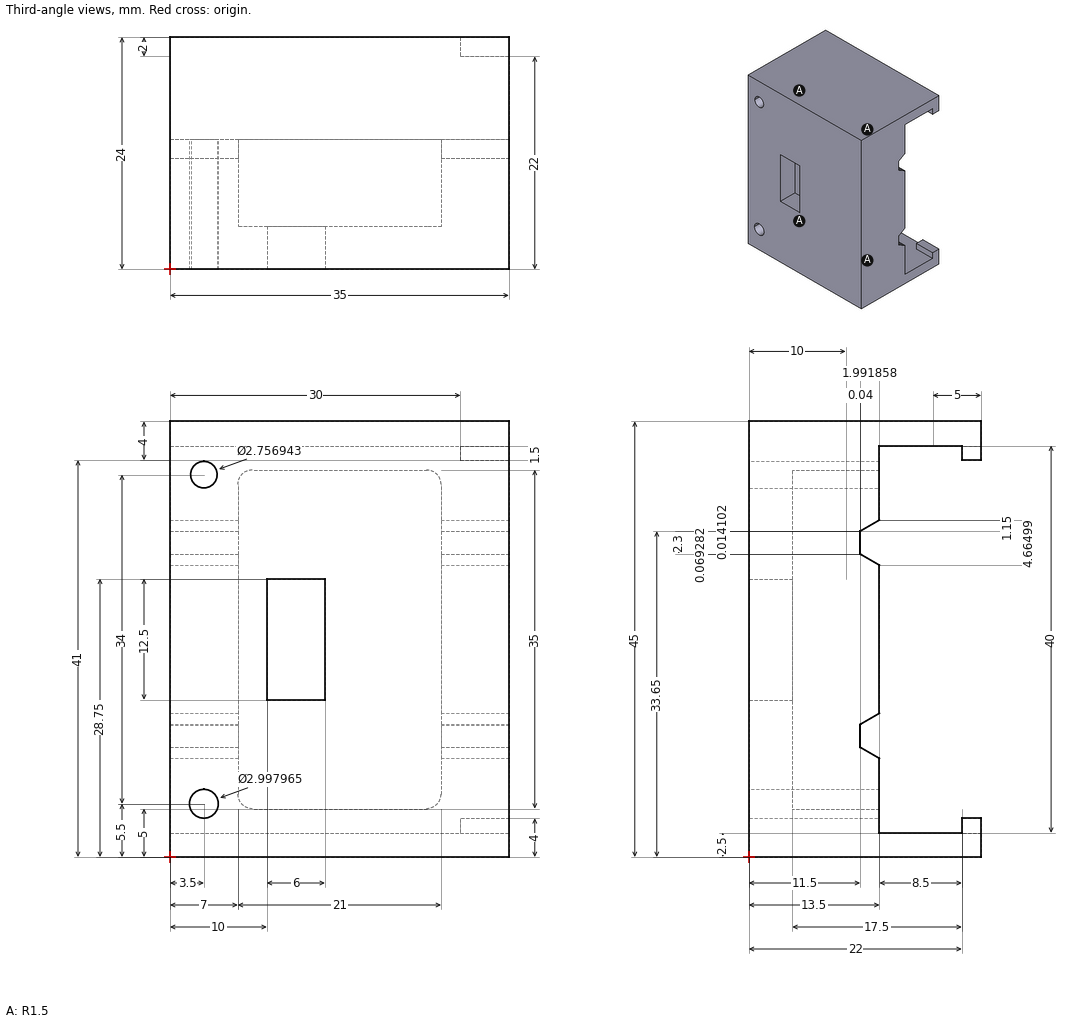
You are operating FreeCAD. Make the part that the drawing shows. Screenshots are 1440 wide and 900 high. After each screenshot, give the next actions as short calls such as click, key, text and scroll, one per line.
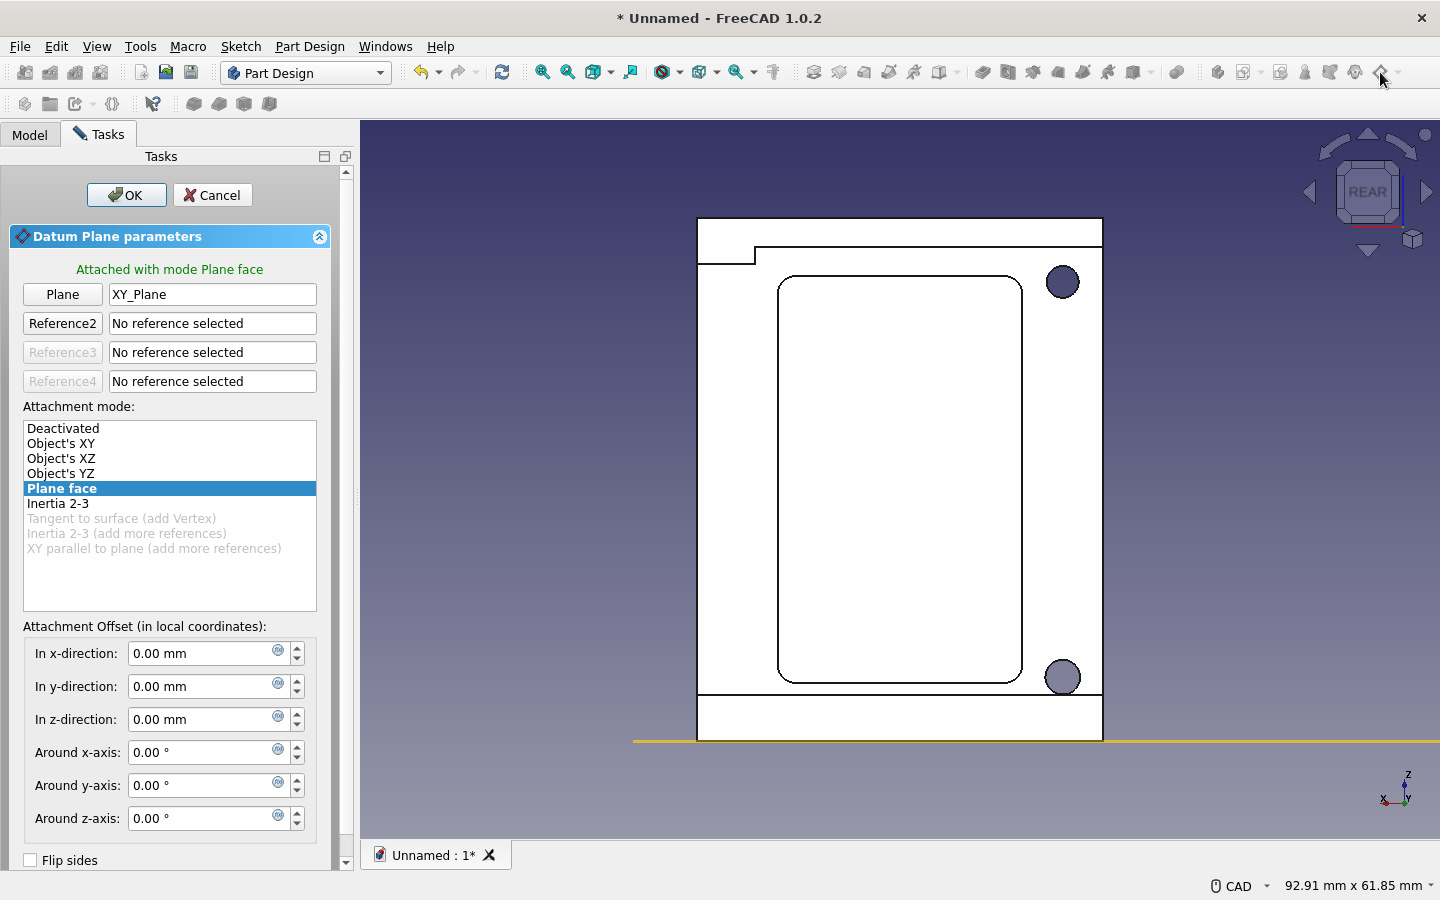
triple_click(210, 720)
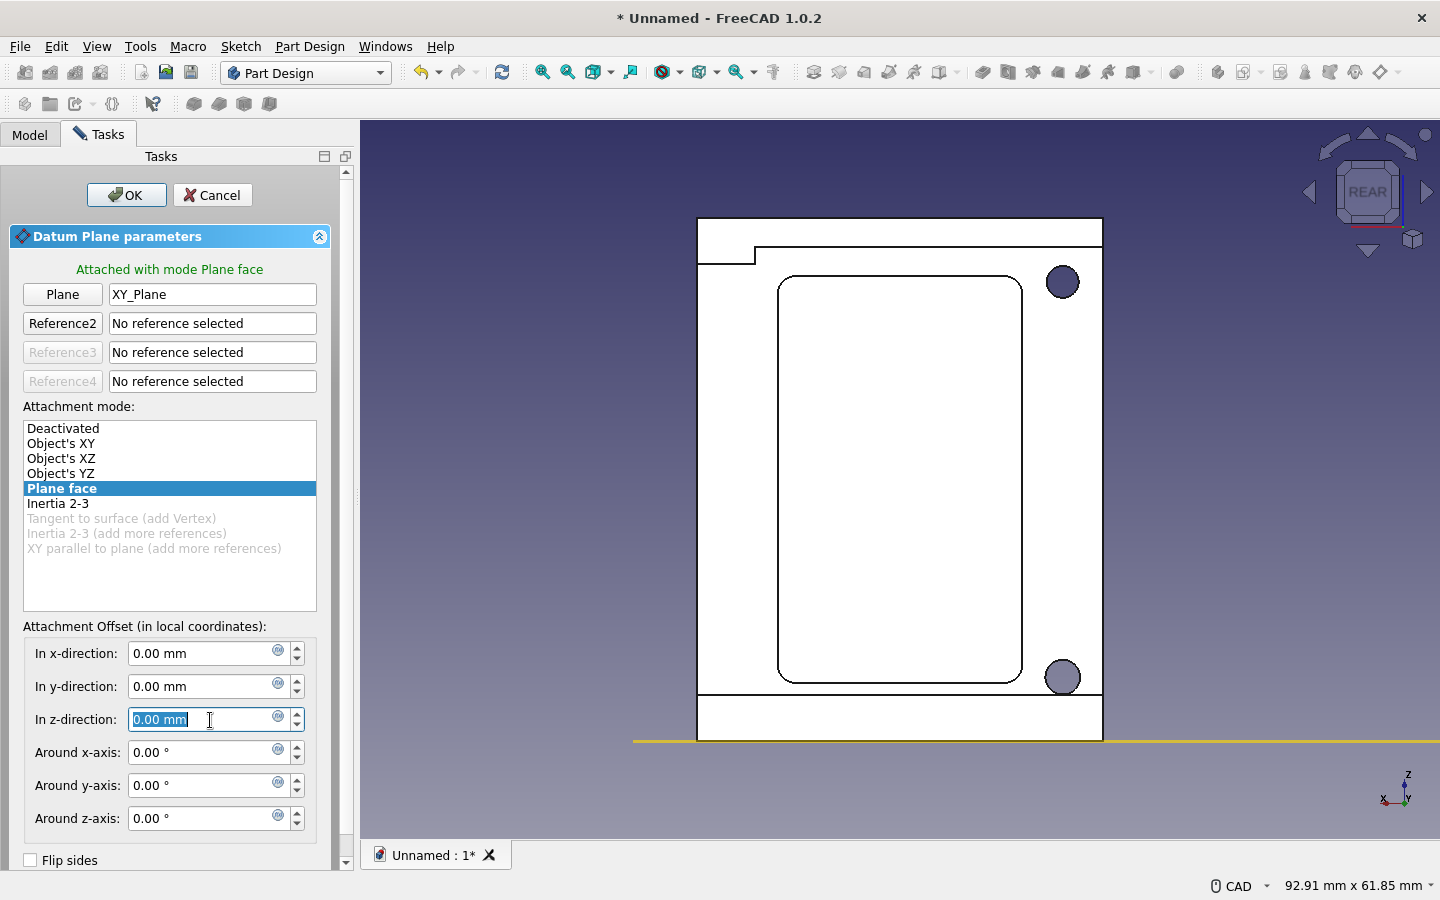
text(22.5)
key(Tab)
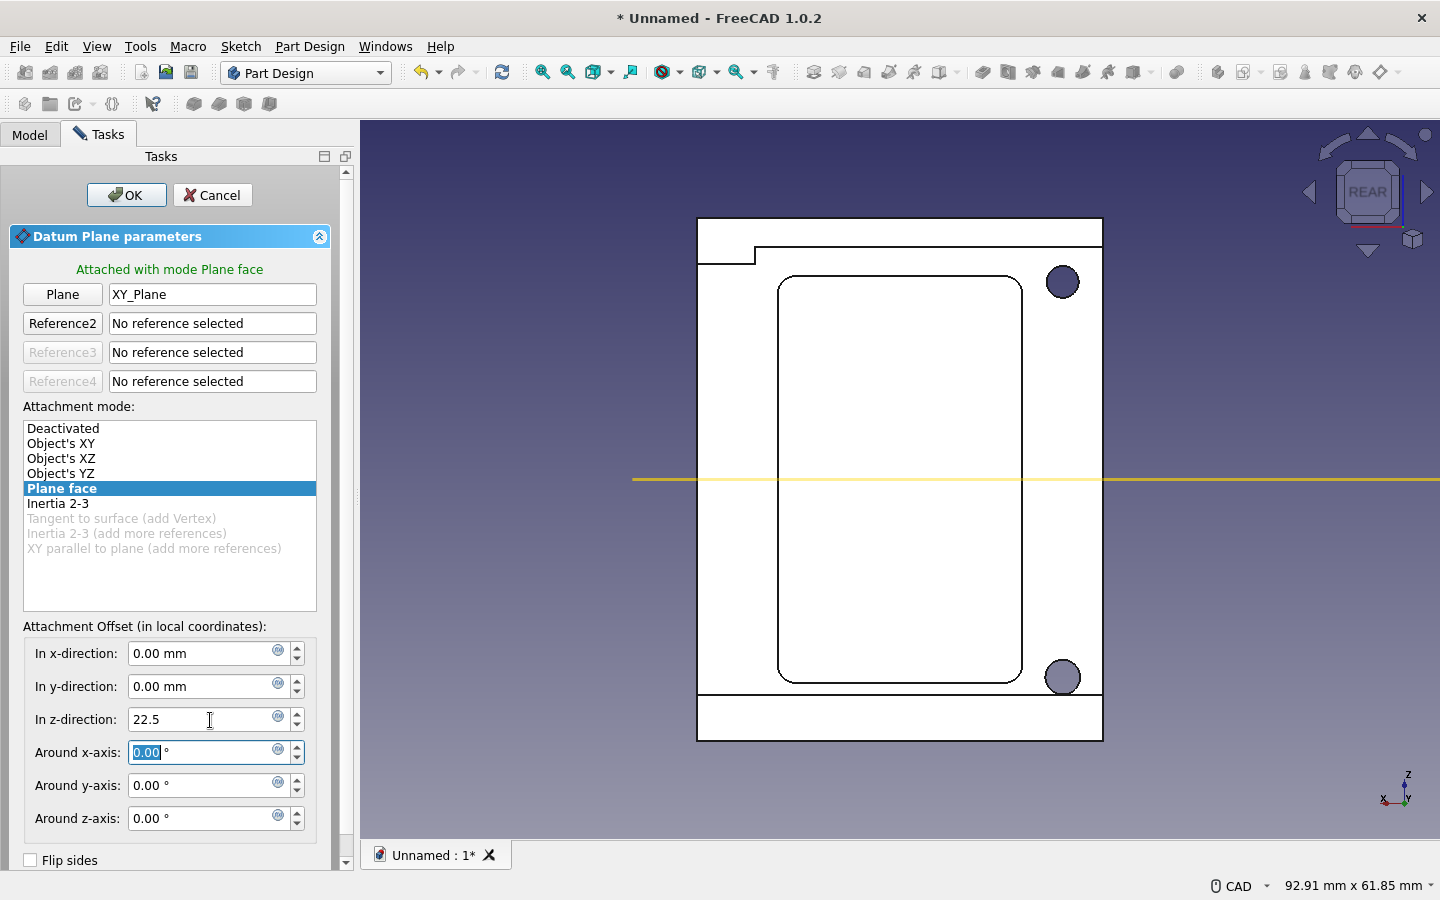
click(127, 195)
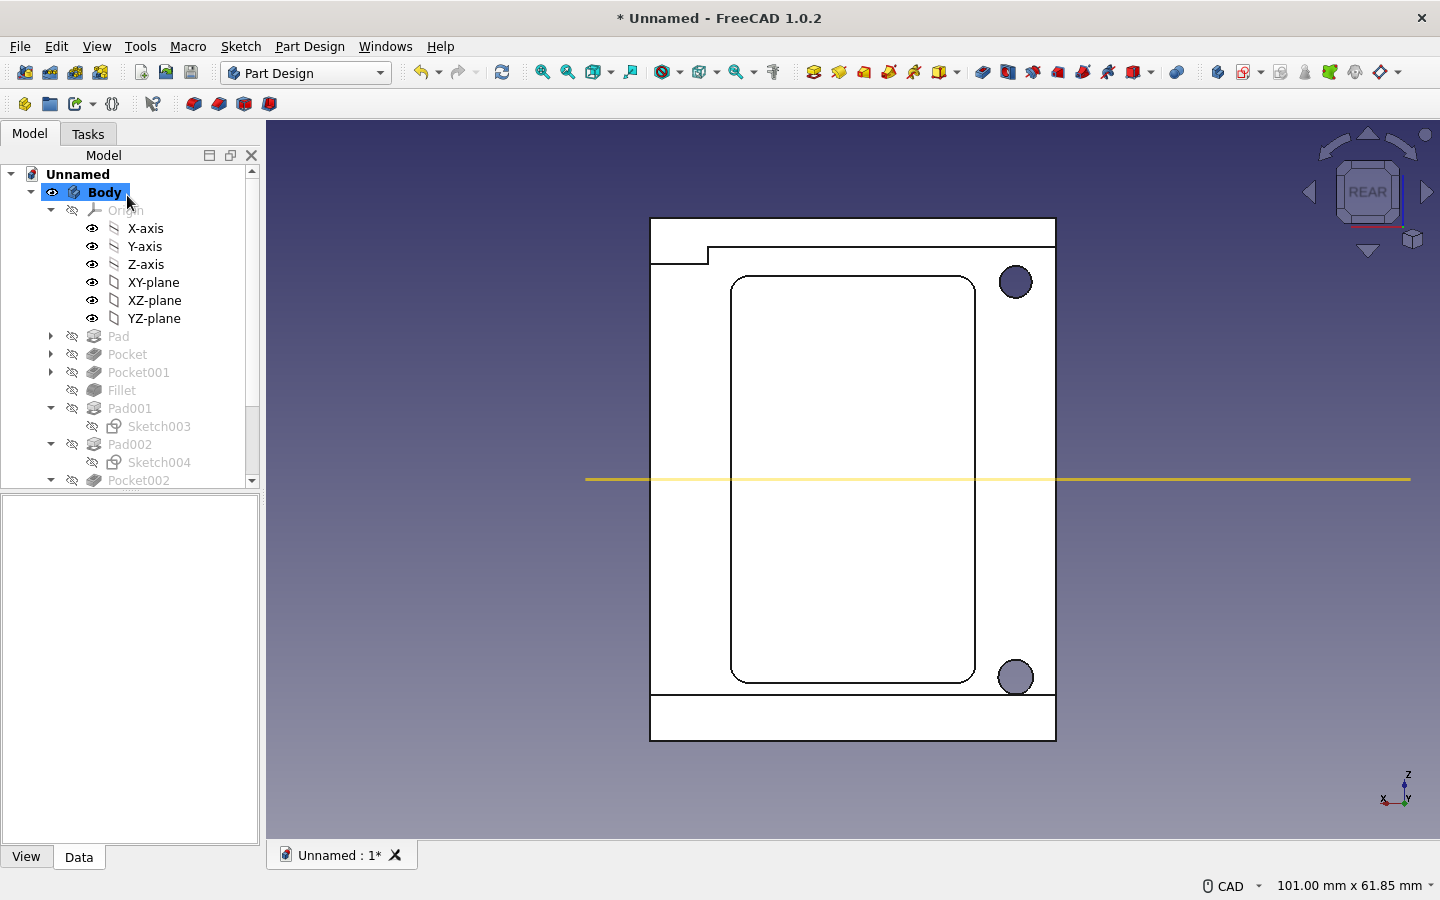
scroll(101, 332, down, 3)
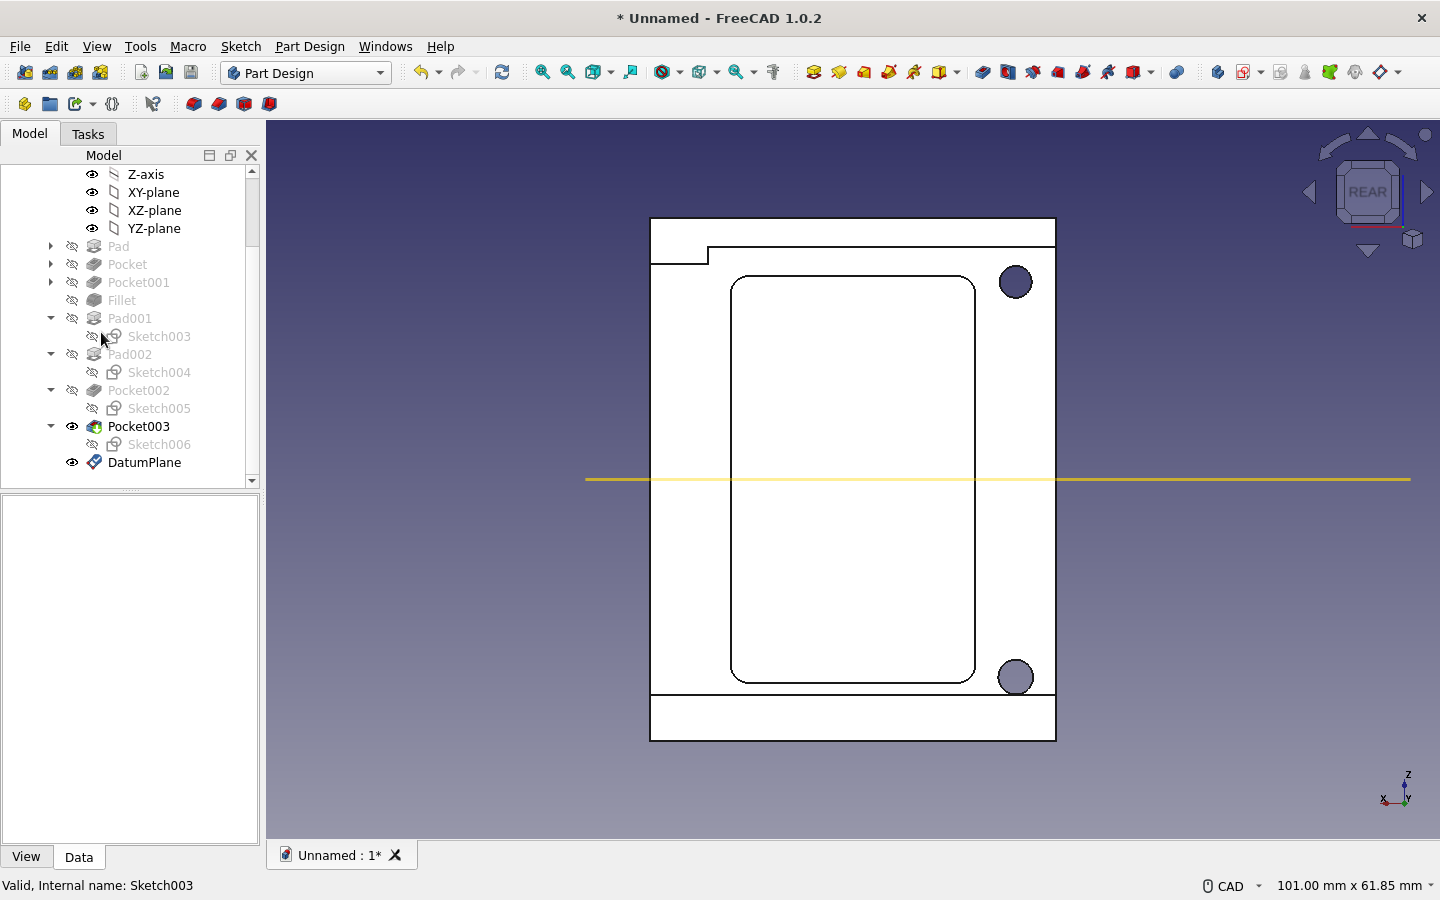
click(117, 426)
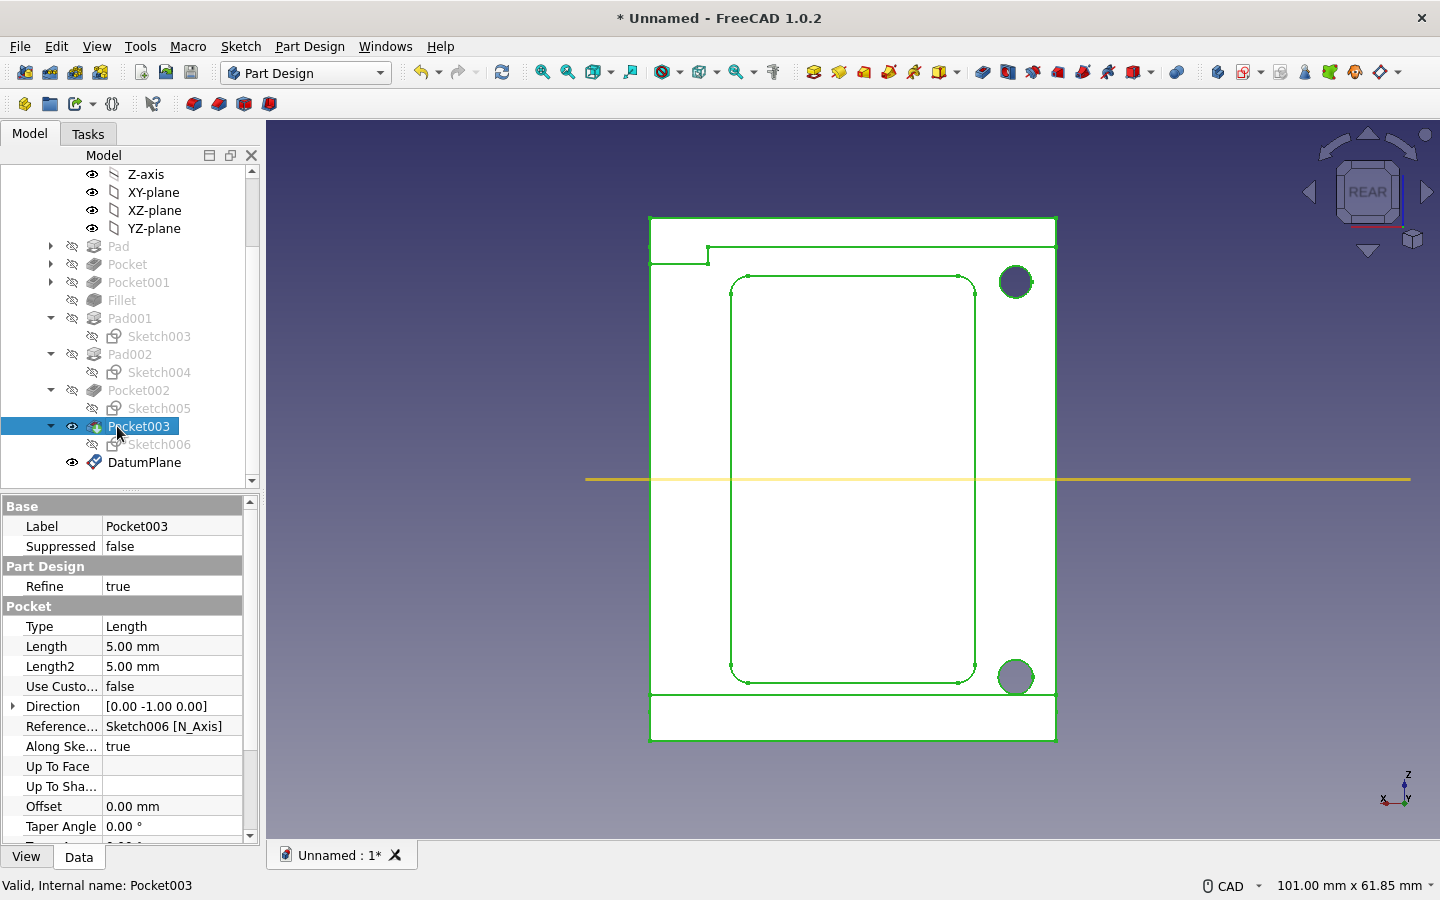
click(25, 72)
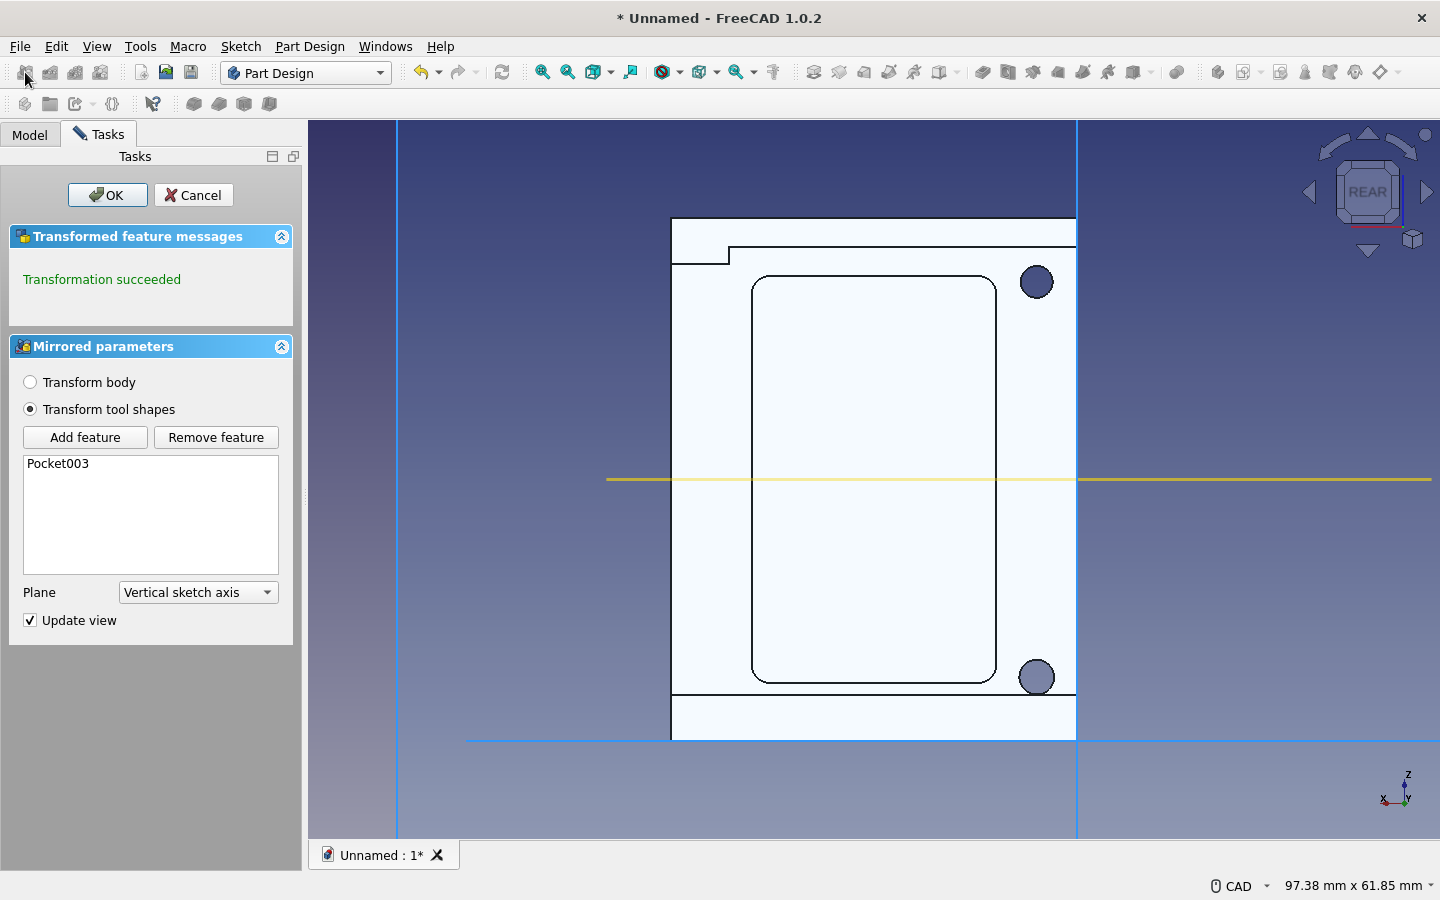
click(199, 592)